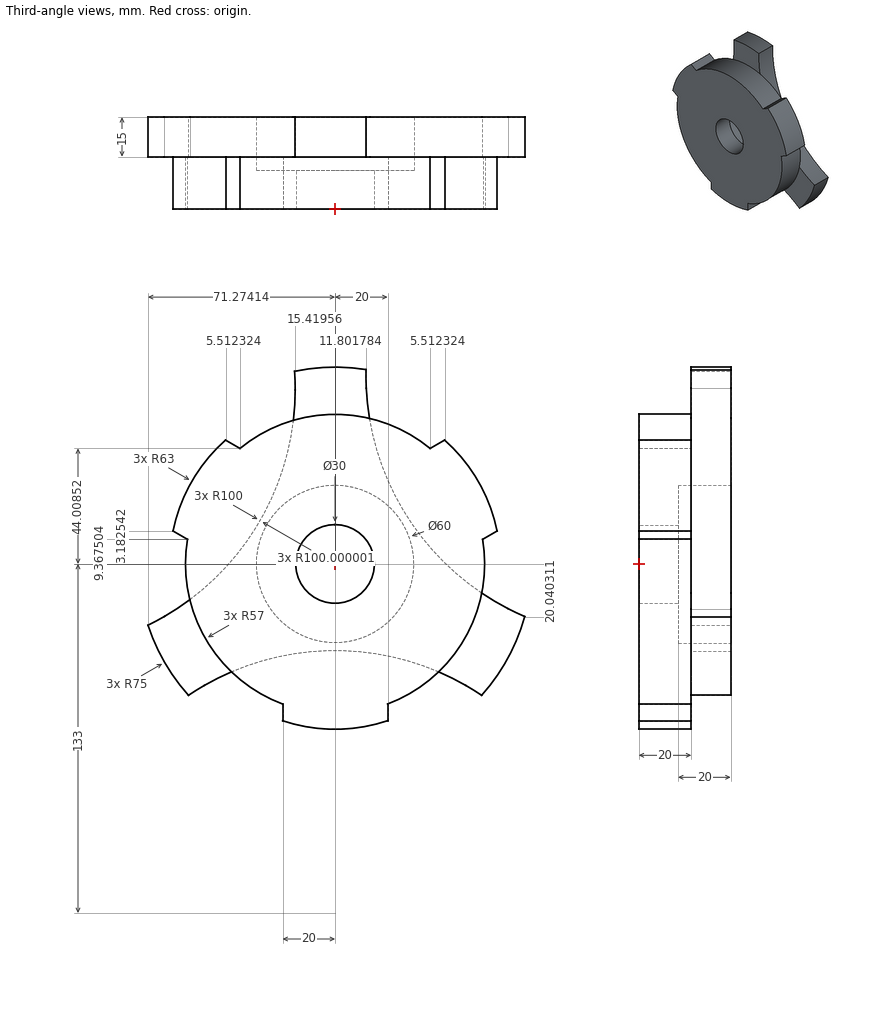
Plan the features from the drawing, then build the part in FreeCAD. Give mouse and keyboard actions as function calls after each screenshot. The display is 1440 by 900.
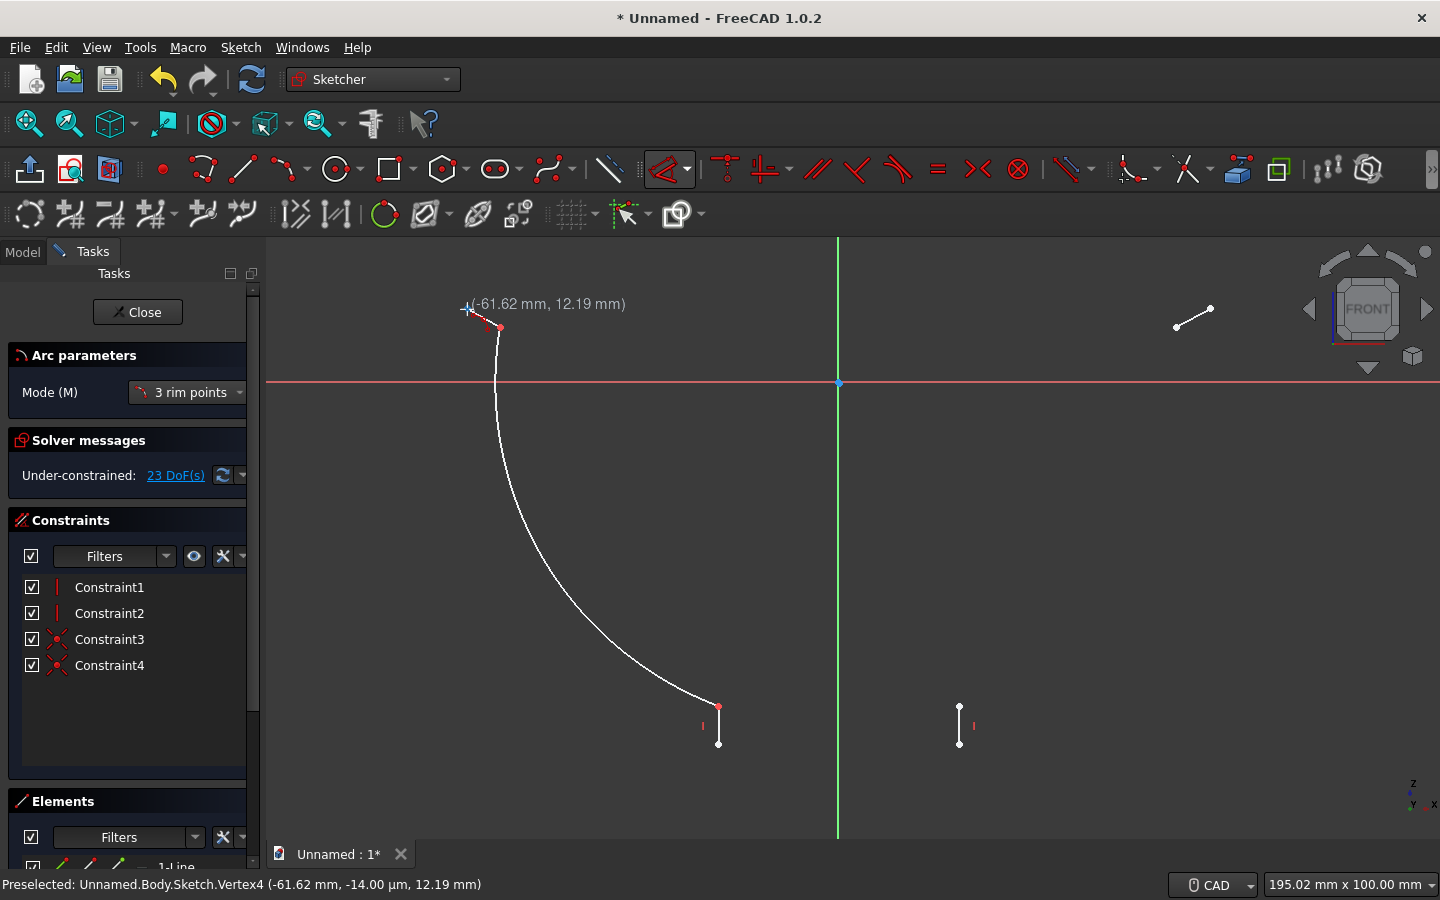
scroll(719, 705, down, 3)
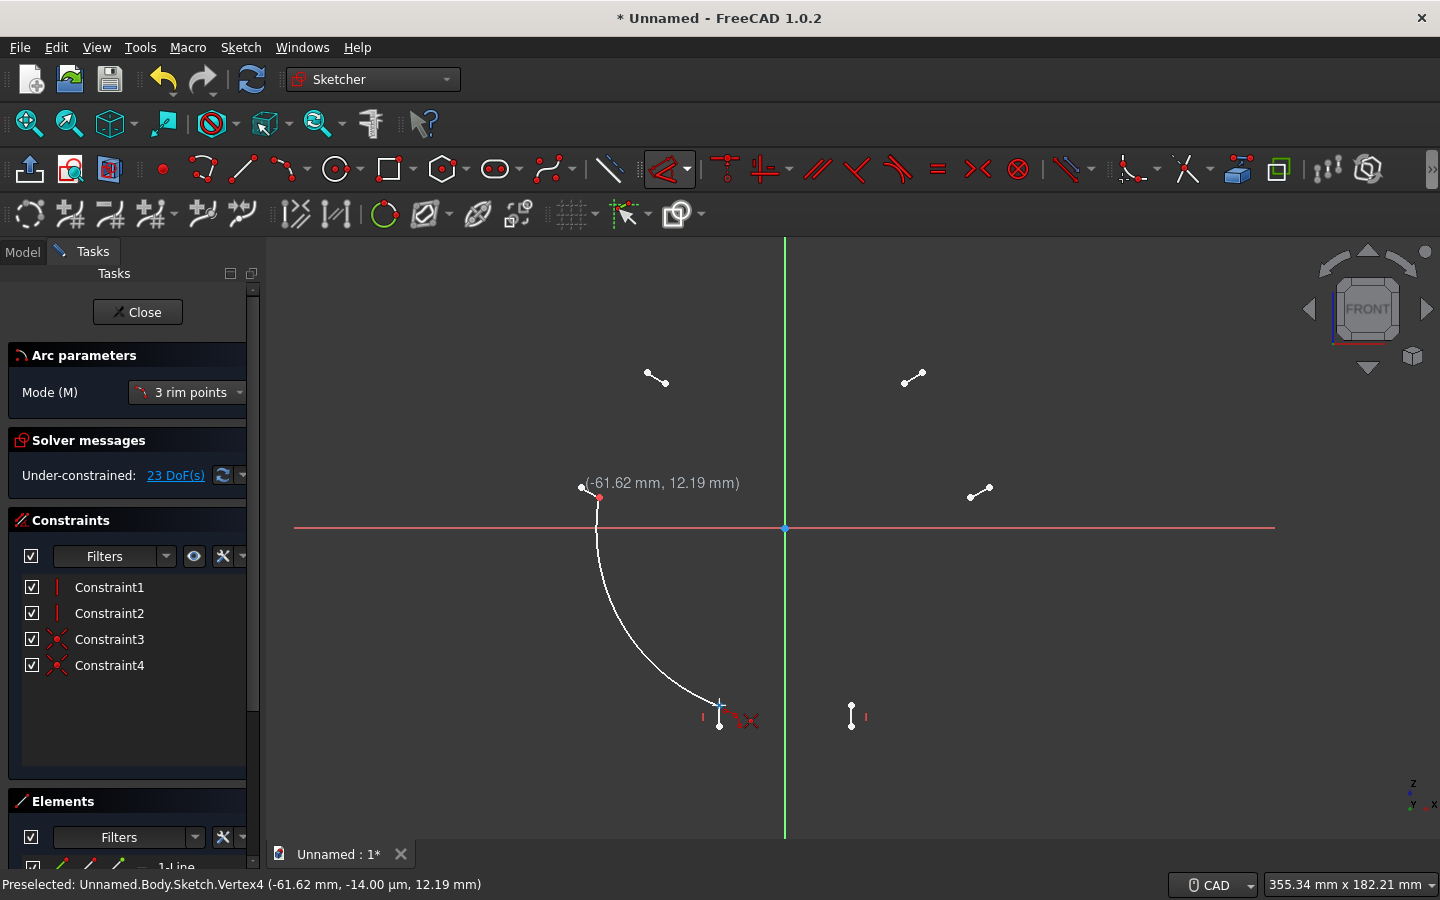
scroll(647, 372, up, 3)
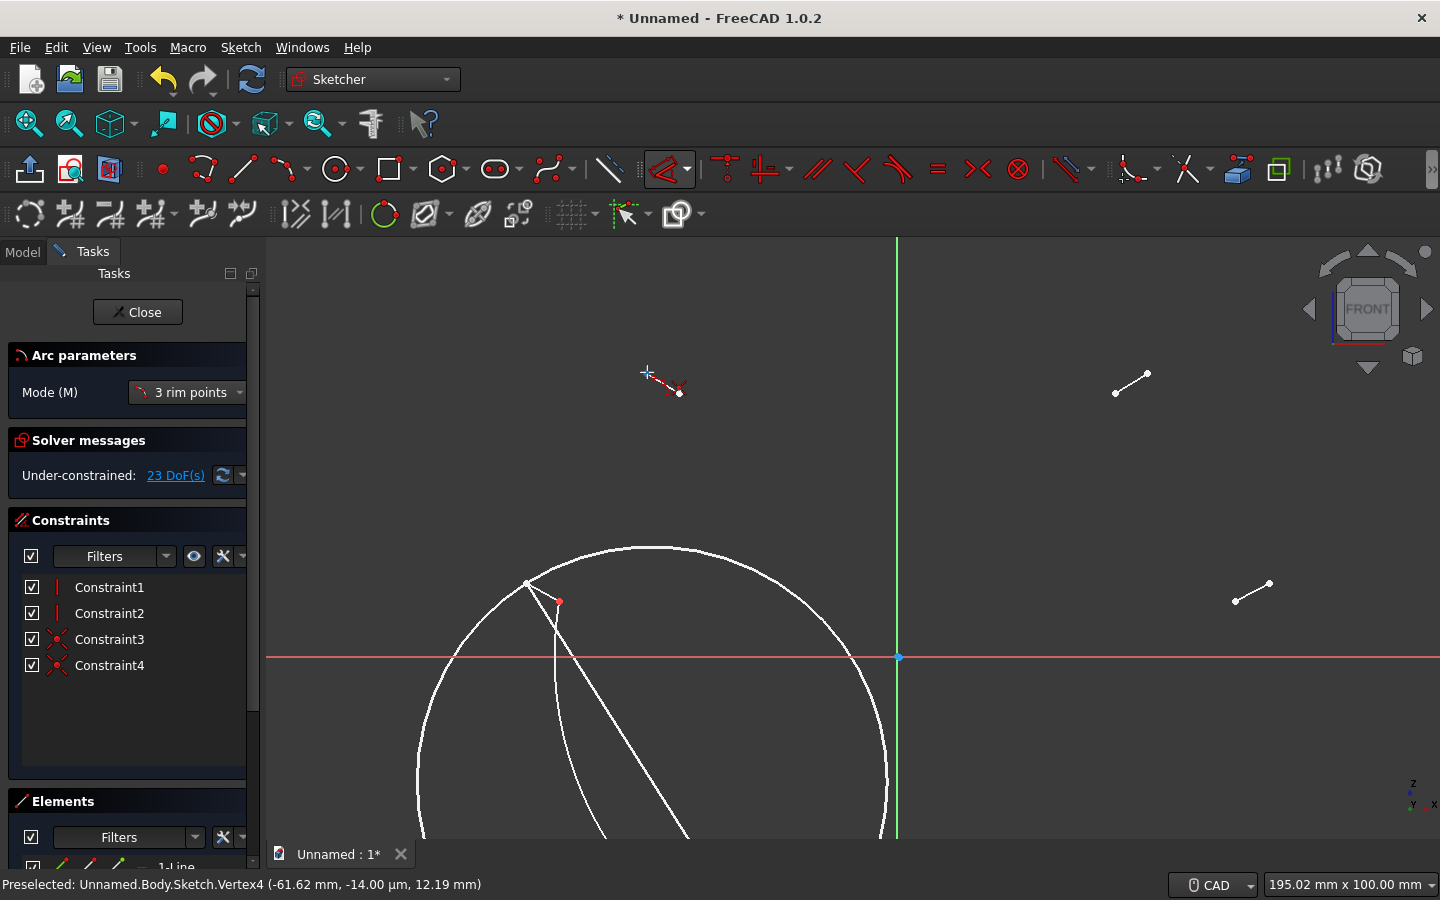
click(647, 374)
click(569, 467)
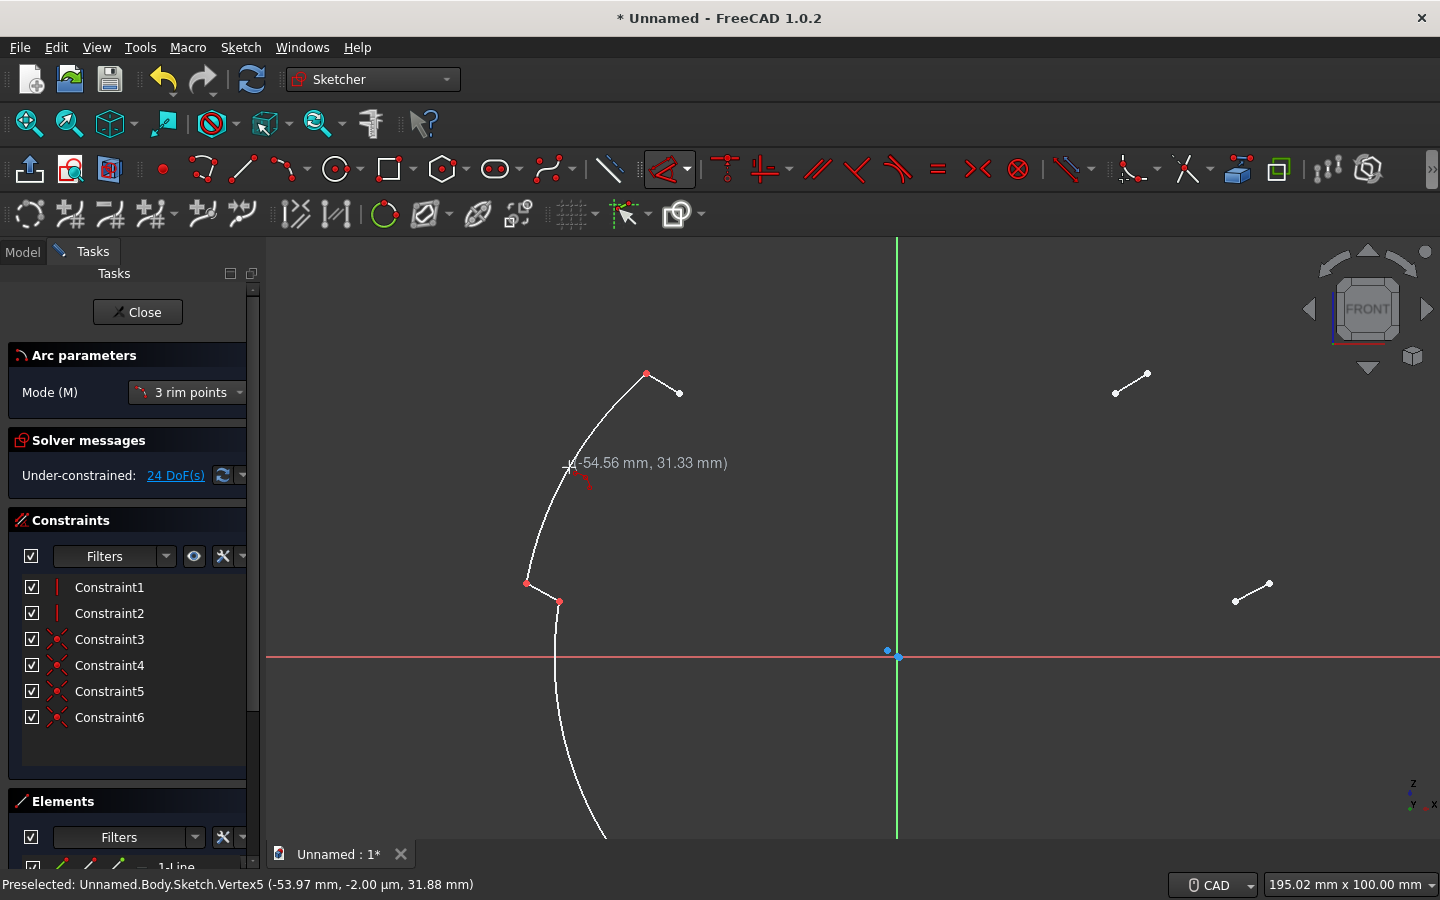
click(680, 394)
click(1115, 394)
click(945, 317)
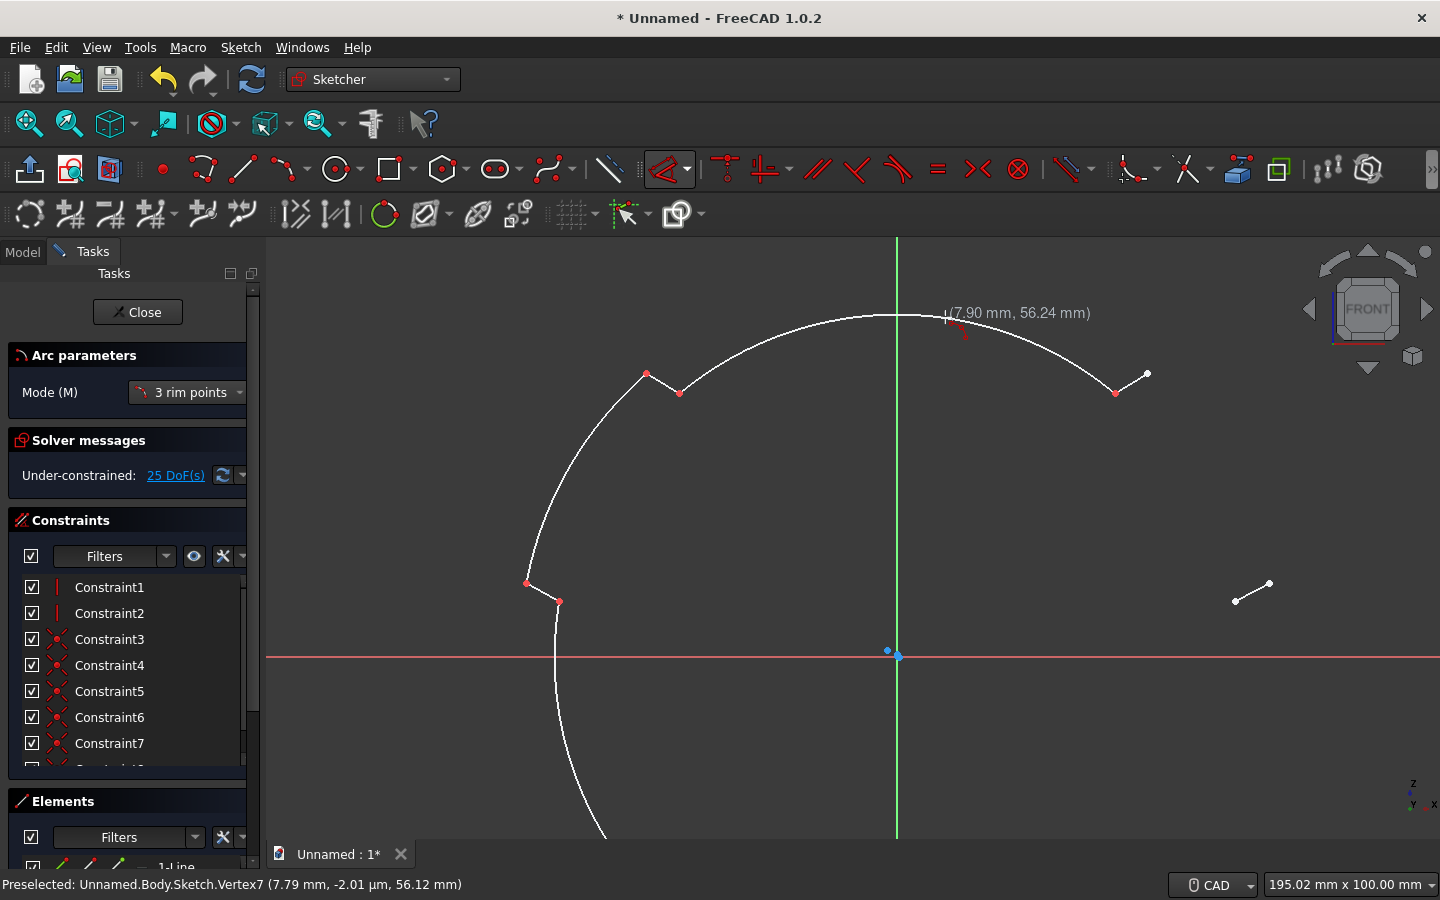
click(1148, 374)
click(1270, 583)
click(1226, 467)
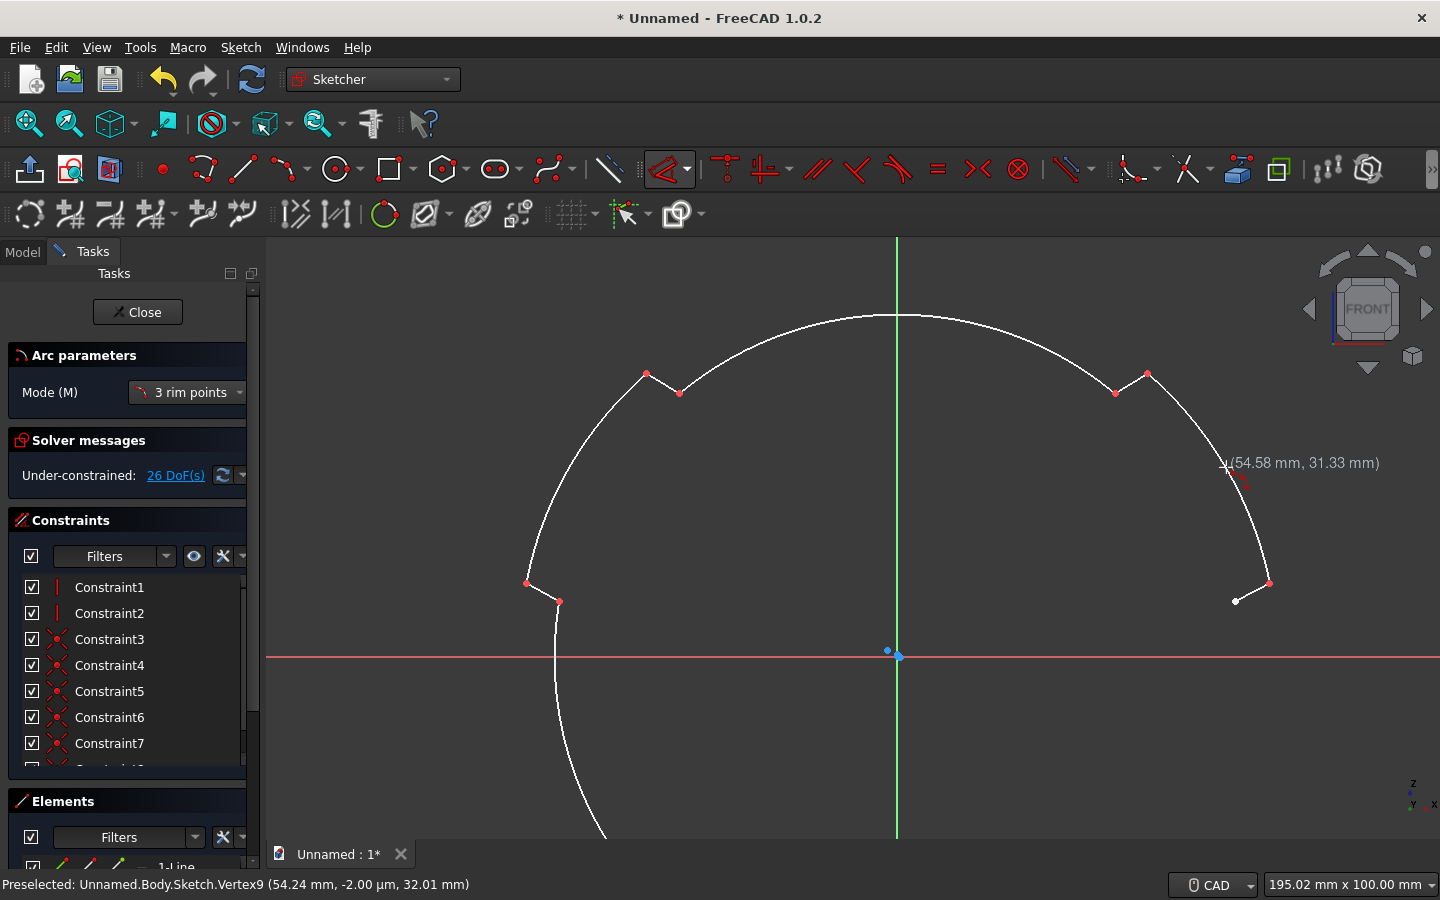
click(1235, 601)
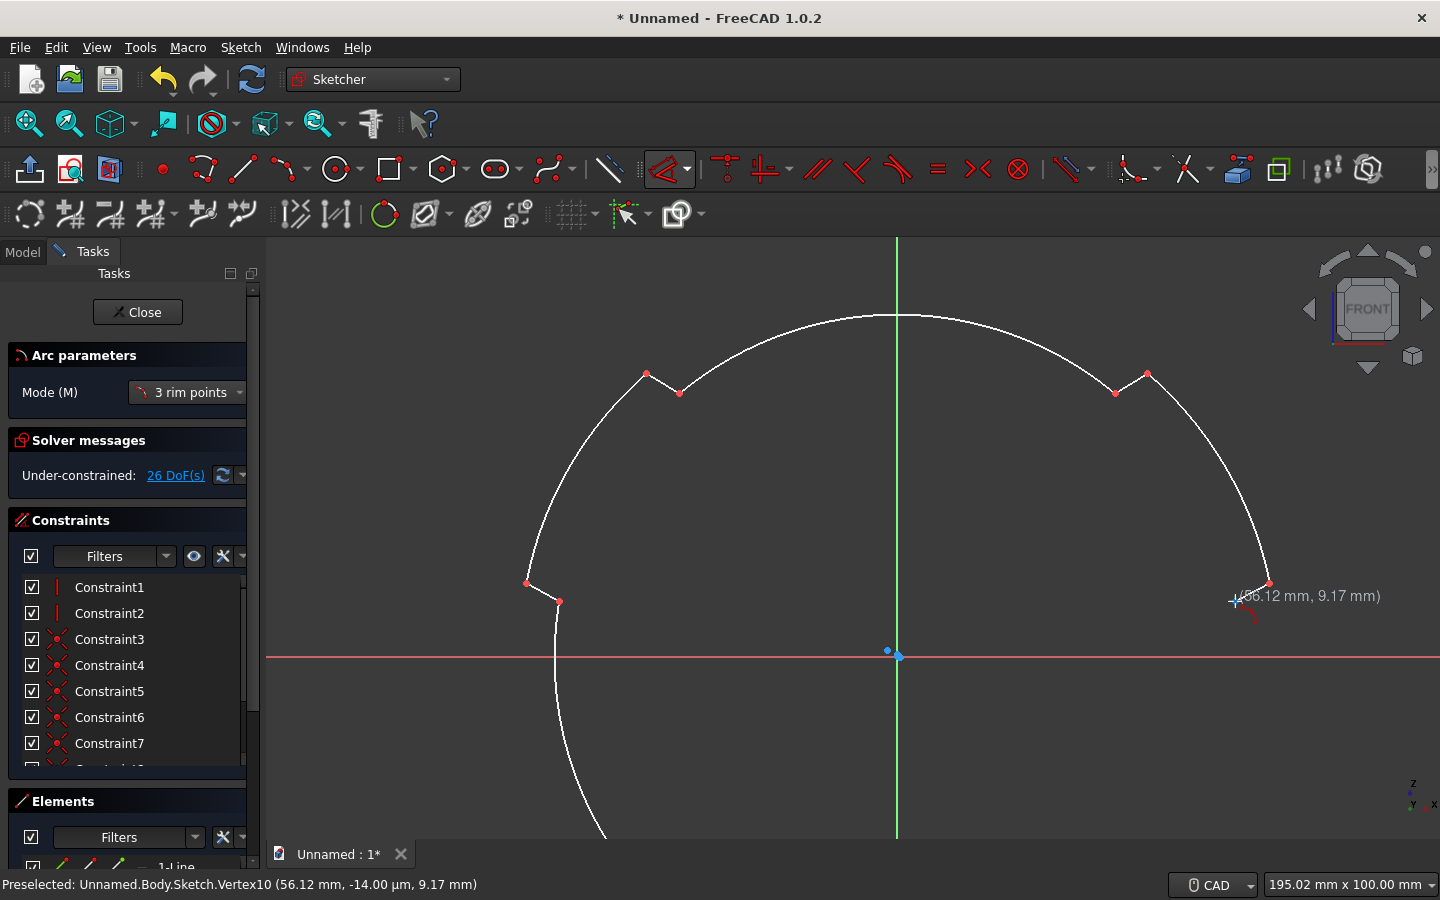
scroll(647, 372, down, 3)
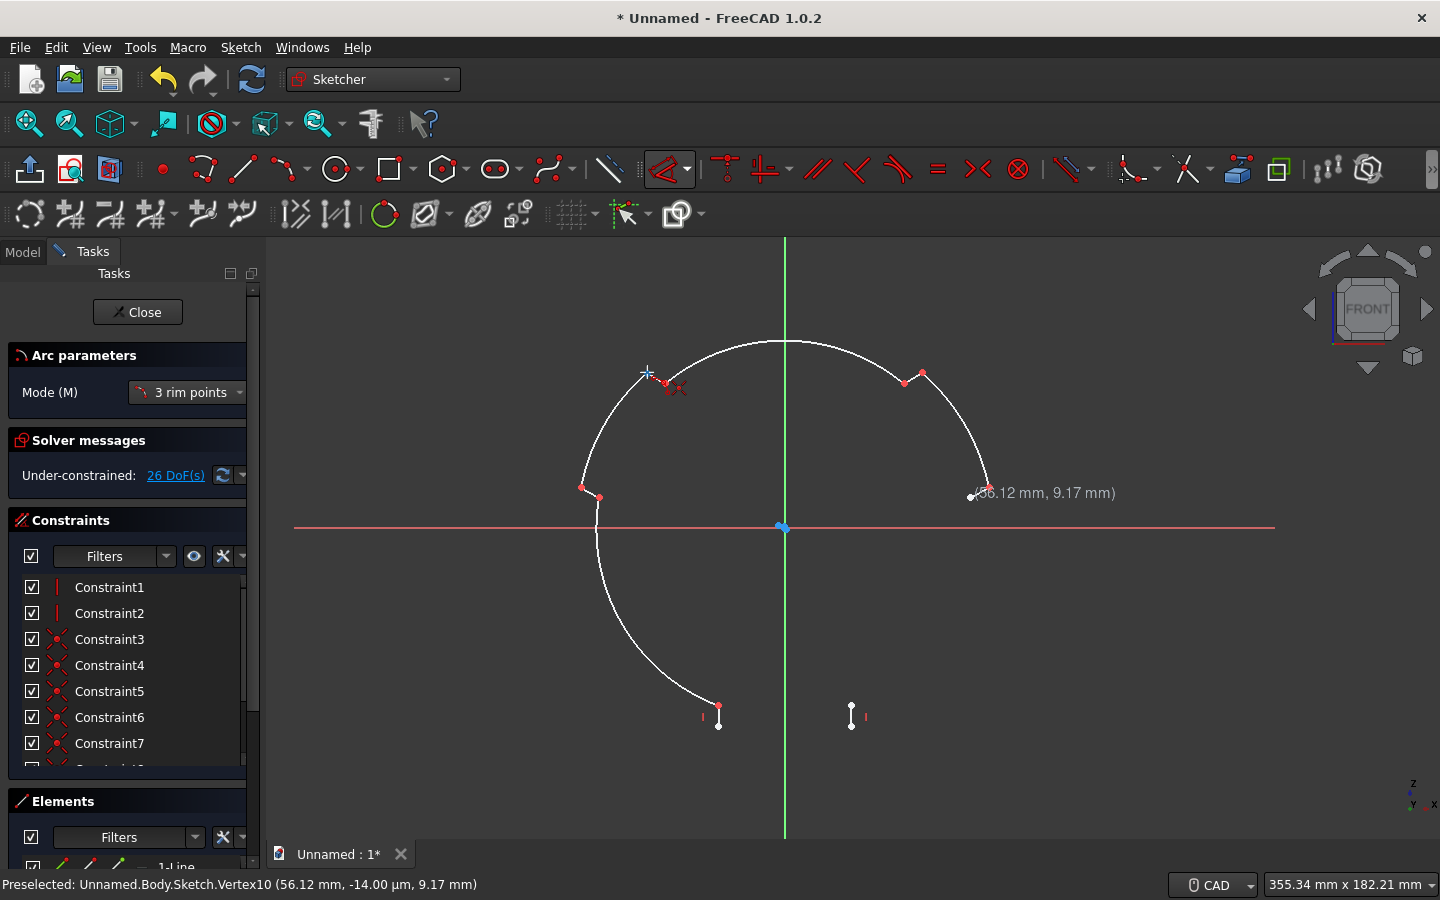
scroll(851, 705, up, 3)